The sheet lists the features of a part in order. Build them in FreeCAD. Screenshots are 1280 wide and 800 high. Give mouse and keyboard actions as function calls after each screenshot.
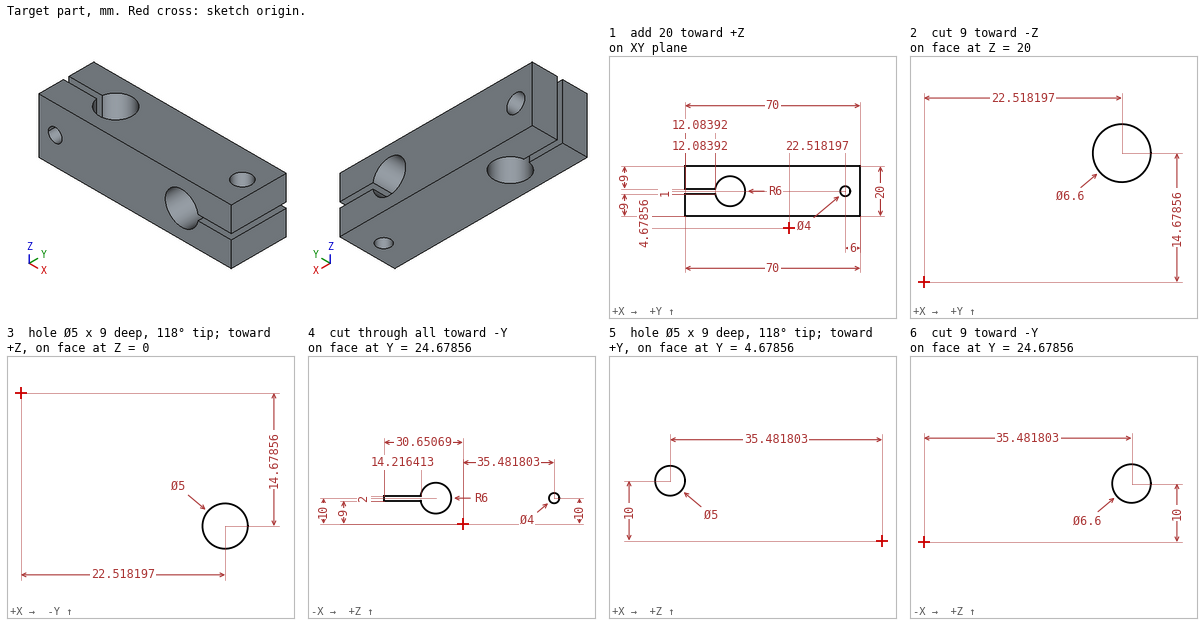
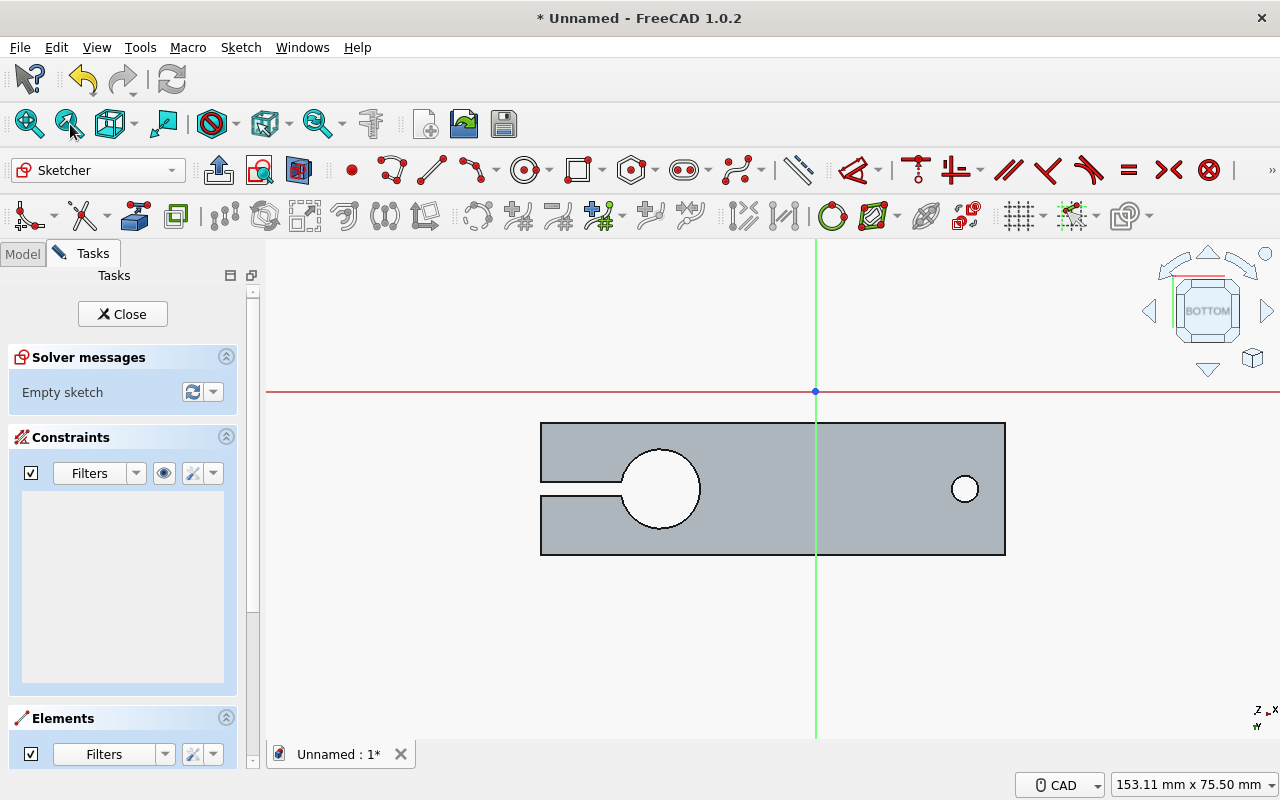
scroll(998, 489, up, 11)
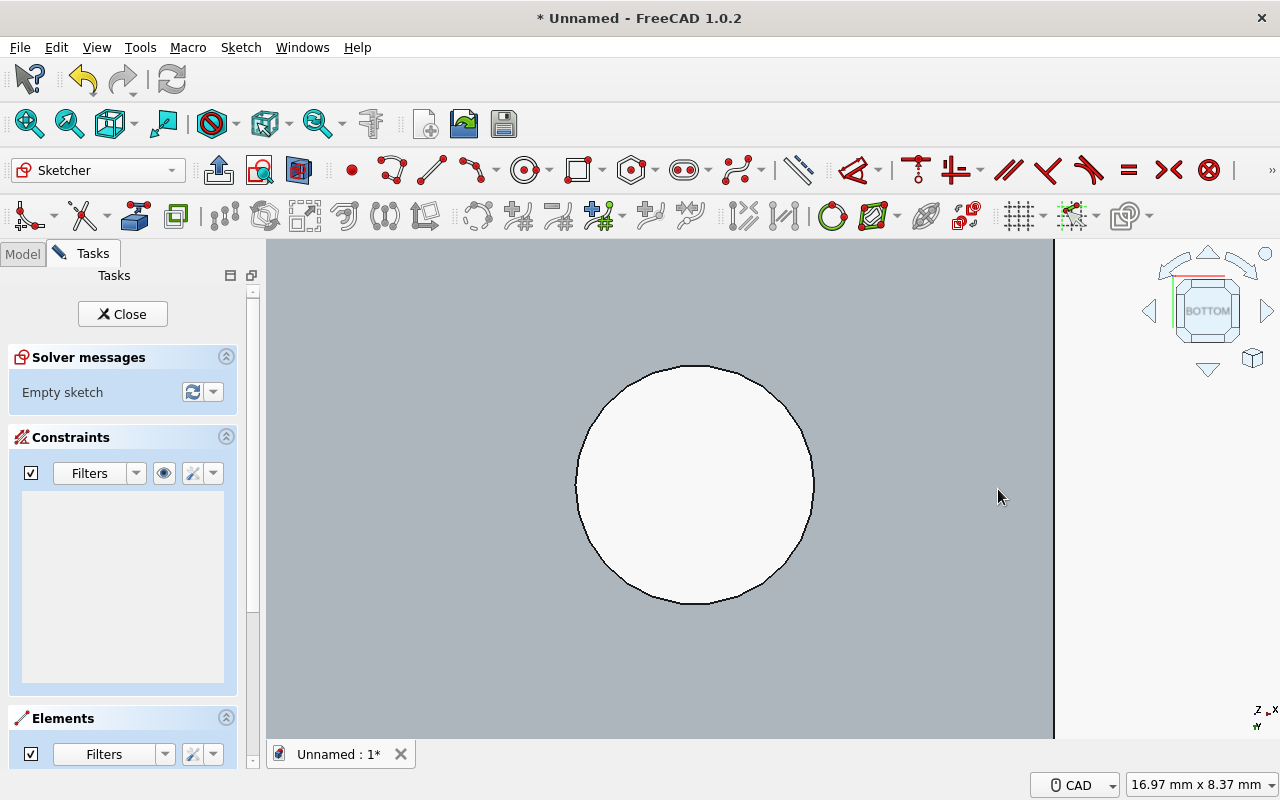
click(526, 170)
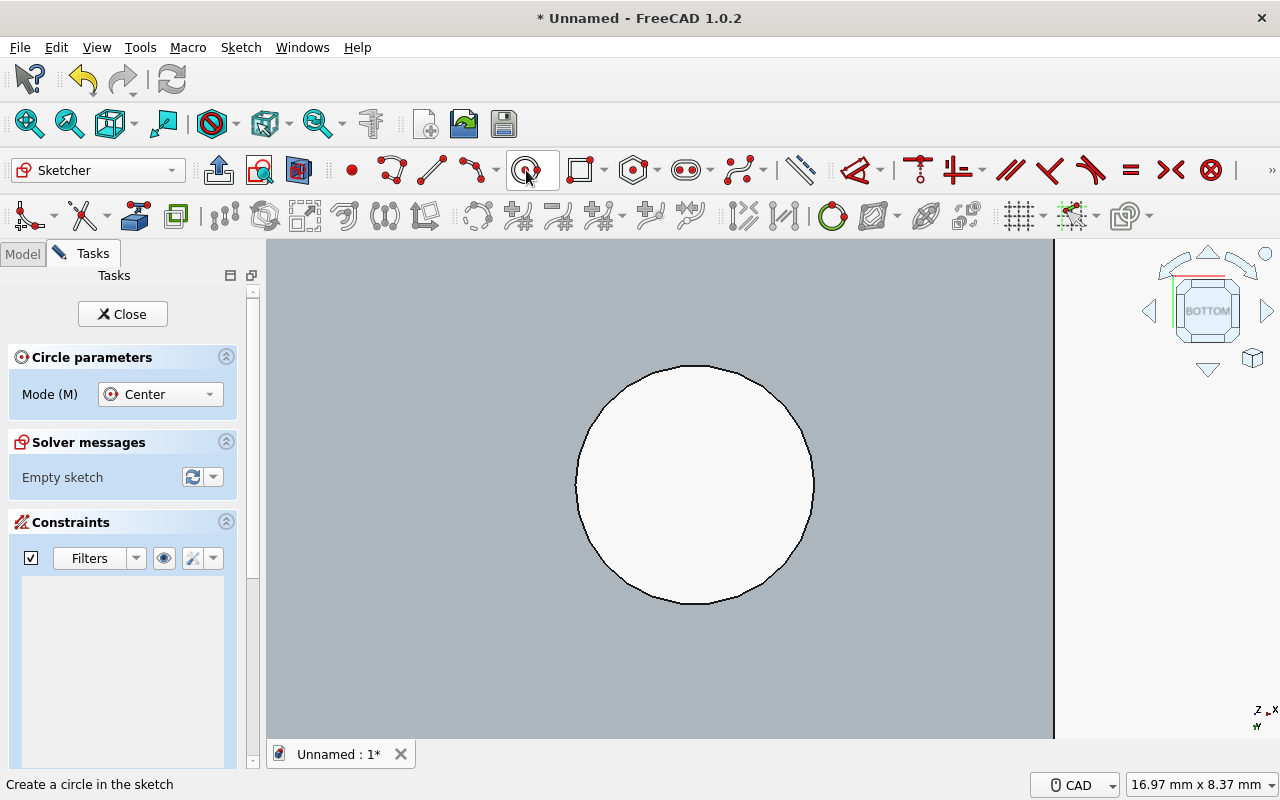
click(695, 485)
click(801, 379)
key(Escape)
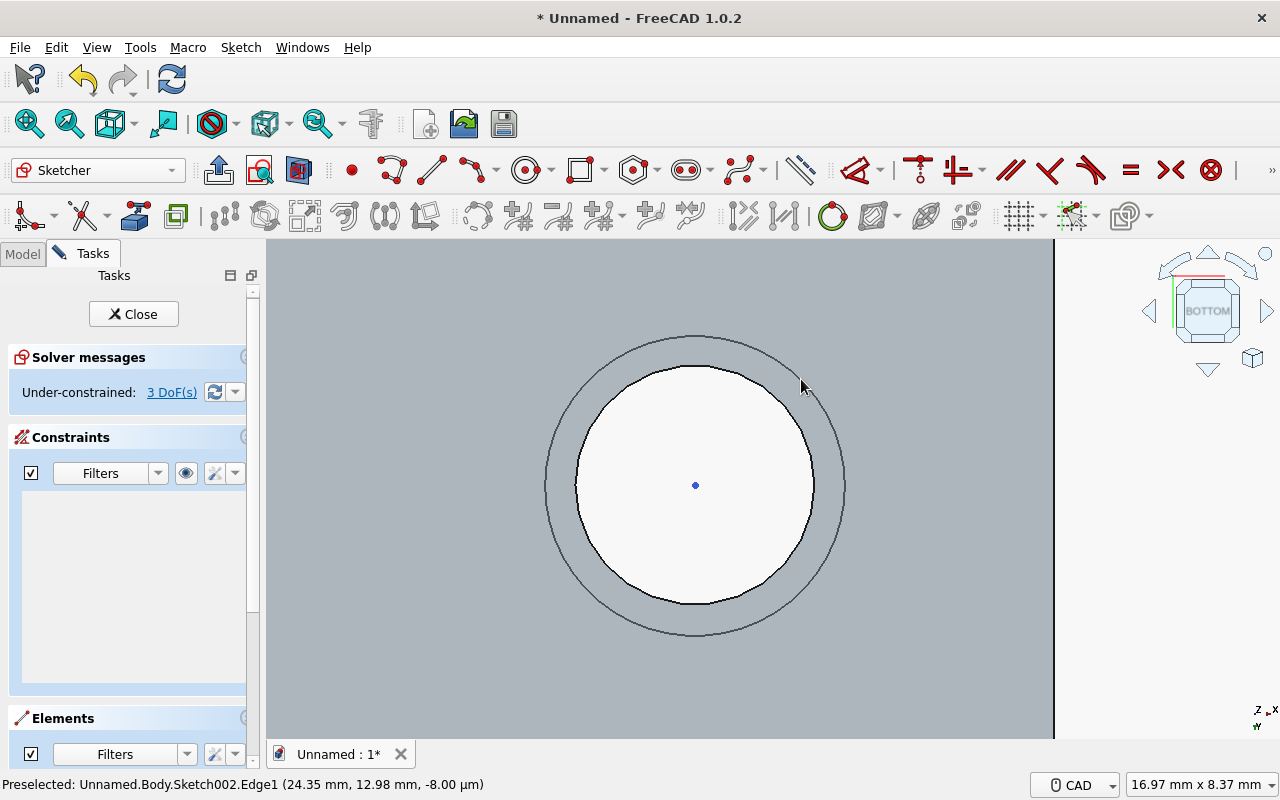
key(d)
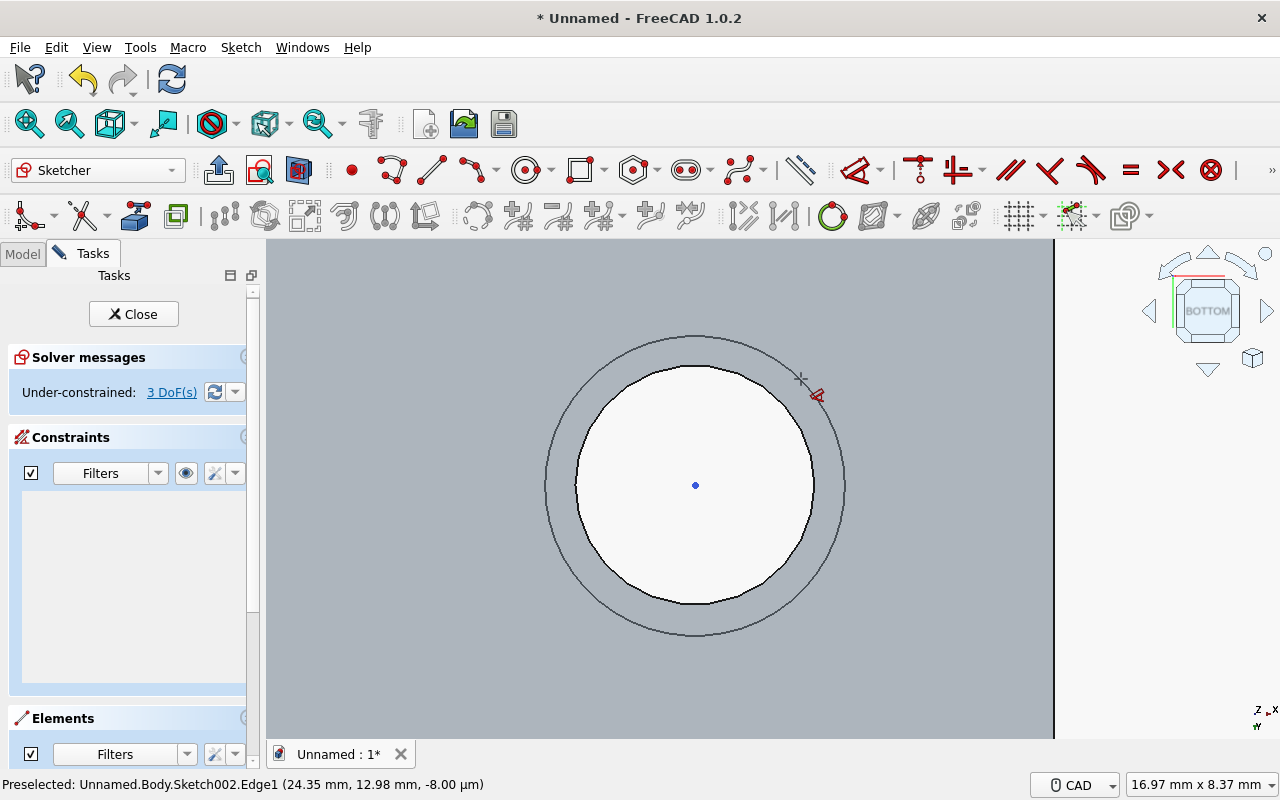
click(801, 380)
click(824, 357)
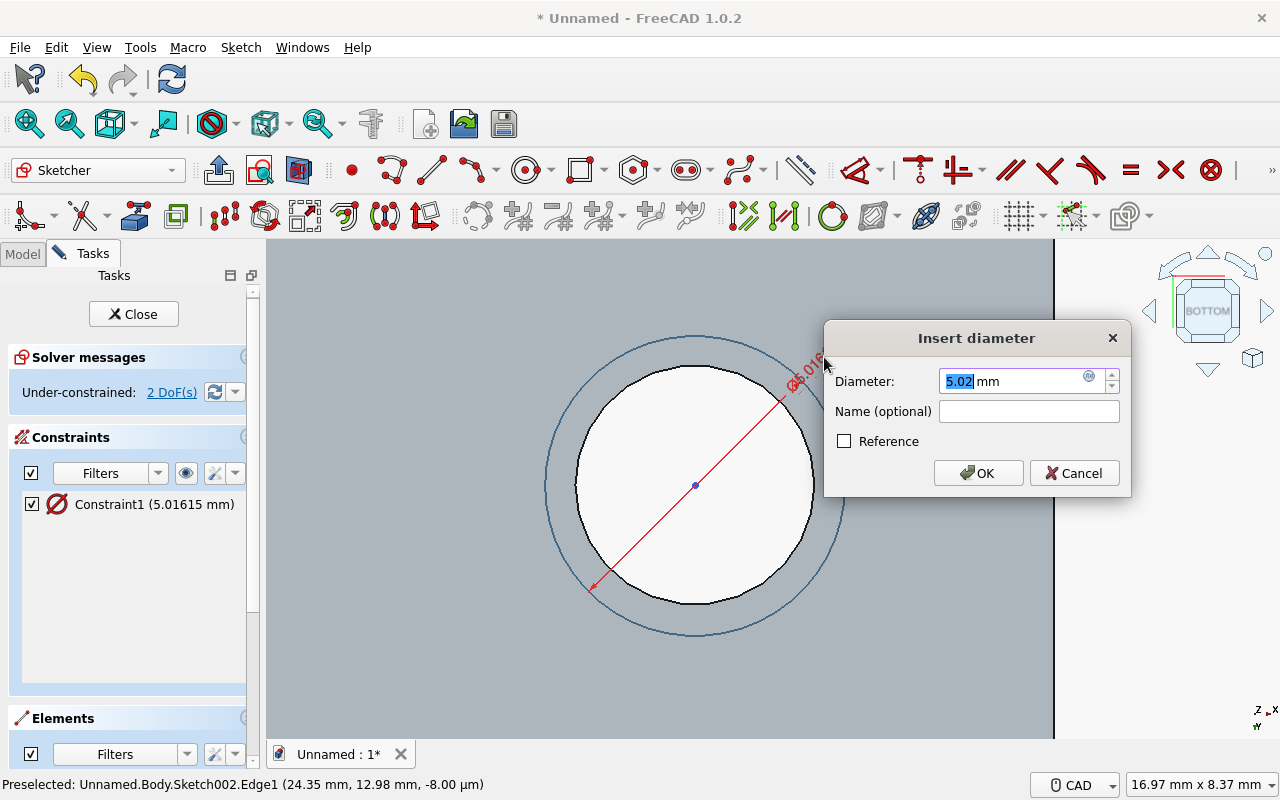
text(5)
key(Return)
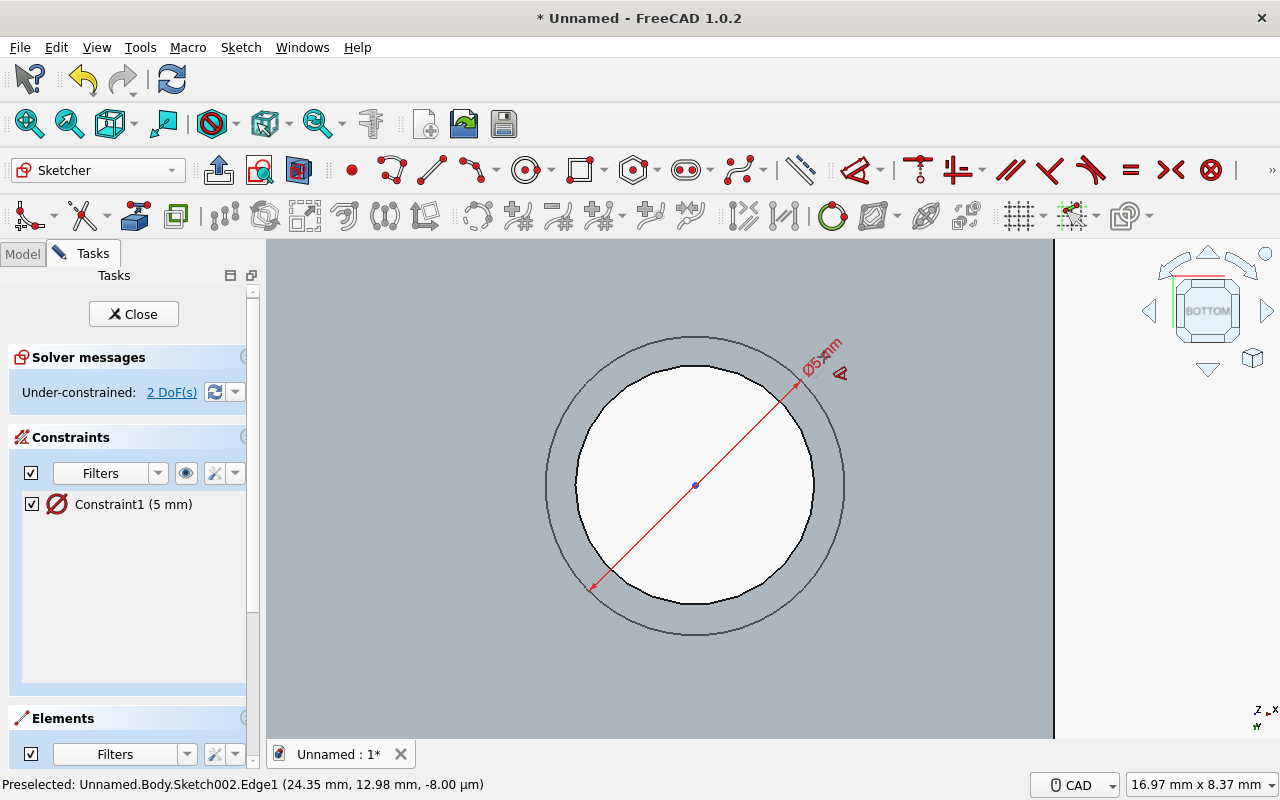
click(695, 486)
click(729, 377)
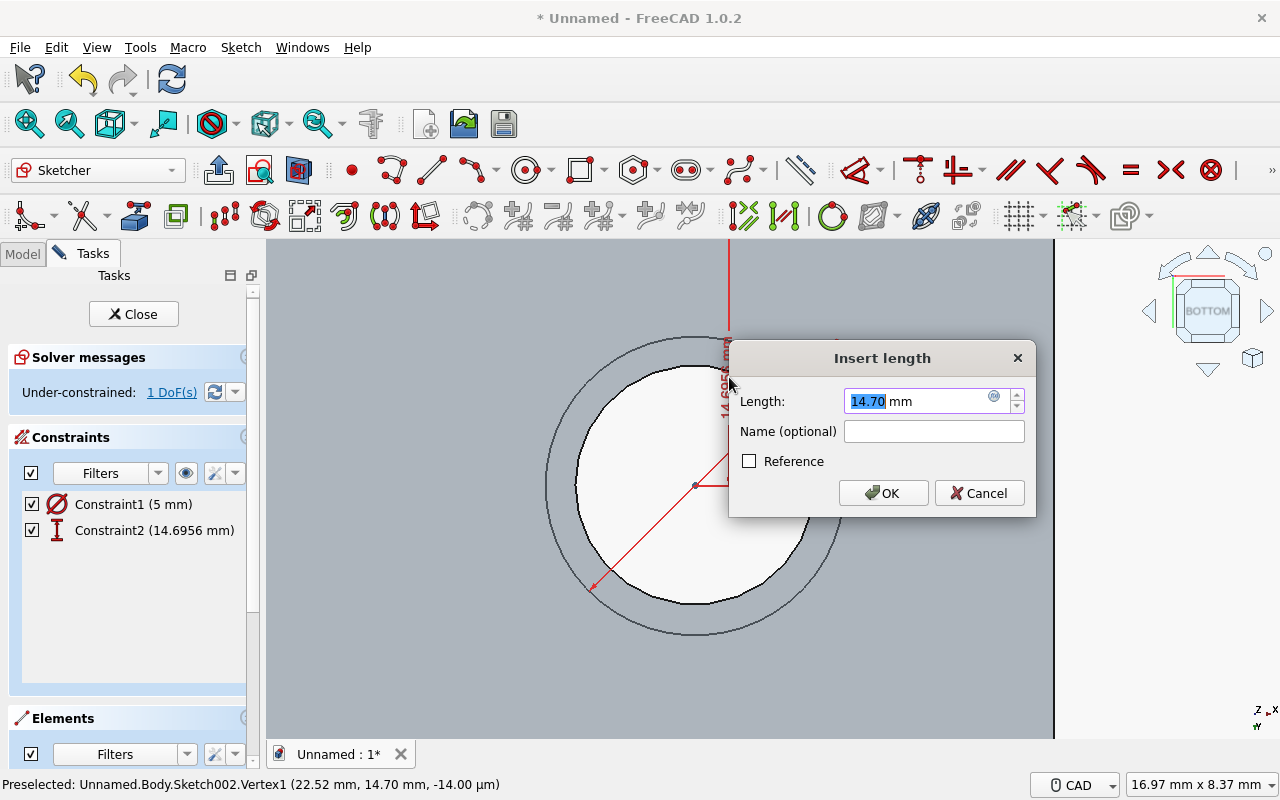
text(14.67856)
key(Return)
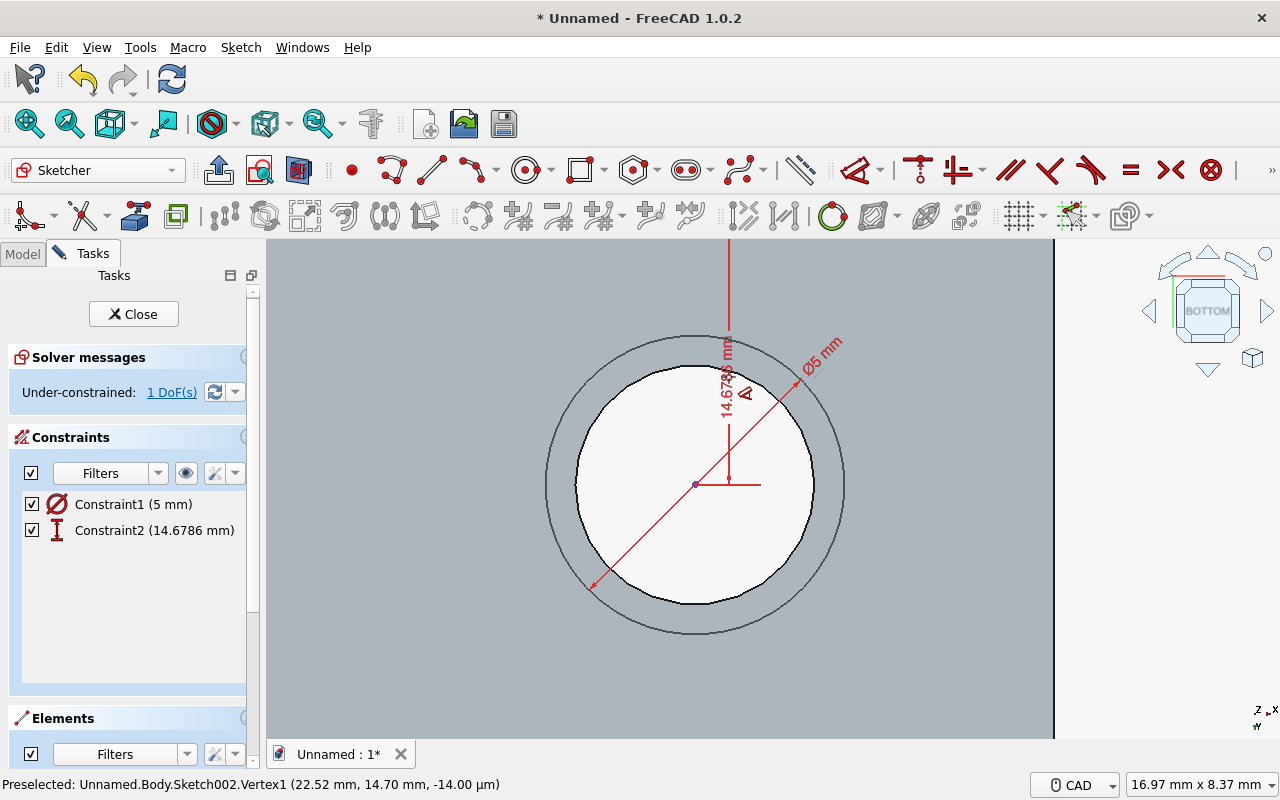
click(695, 485)
click(494, 519)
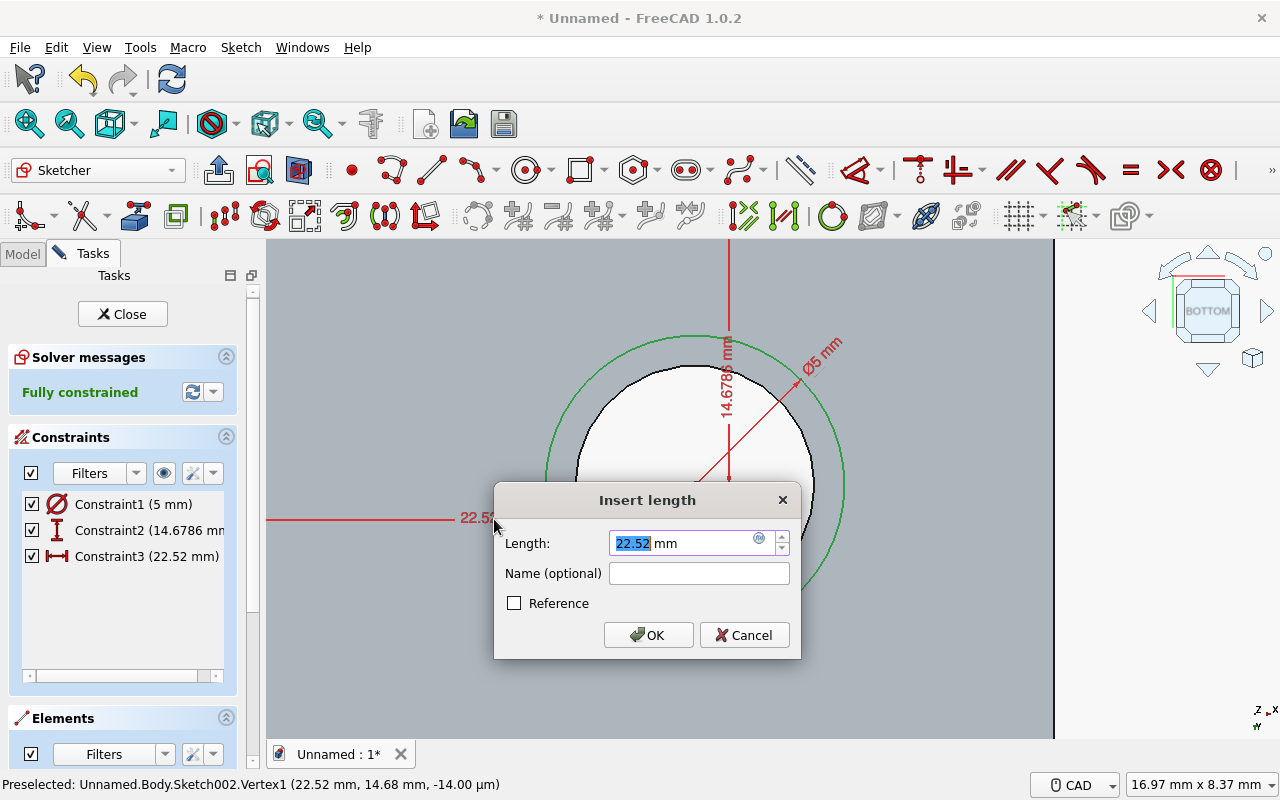
text(22.518197)
key(Return)
key(Escape)